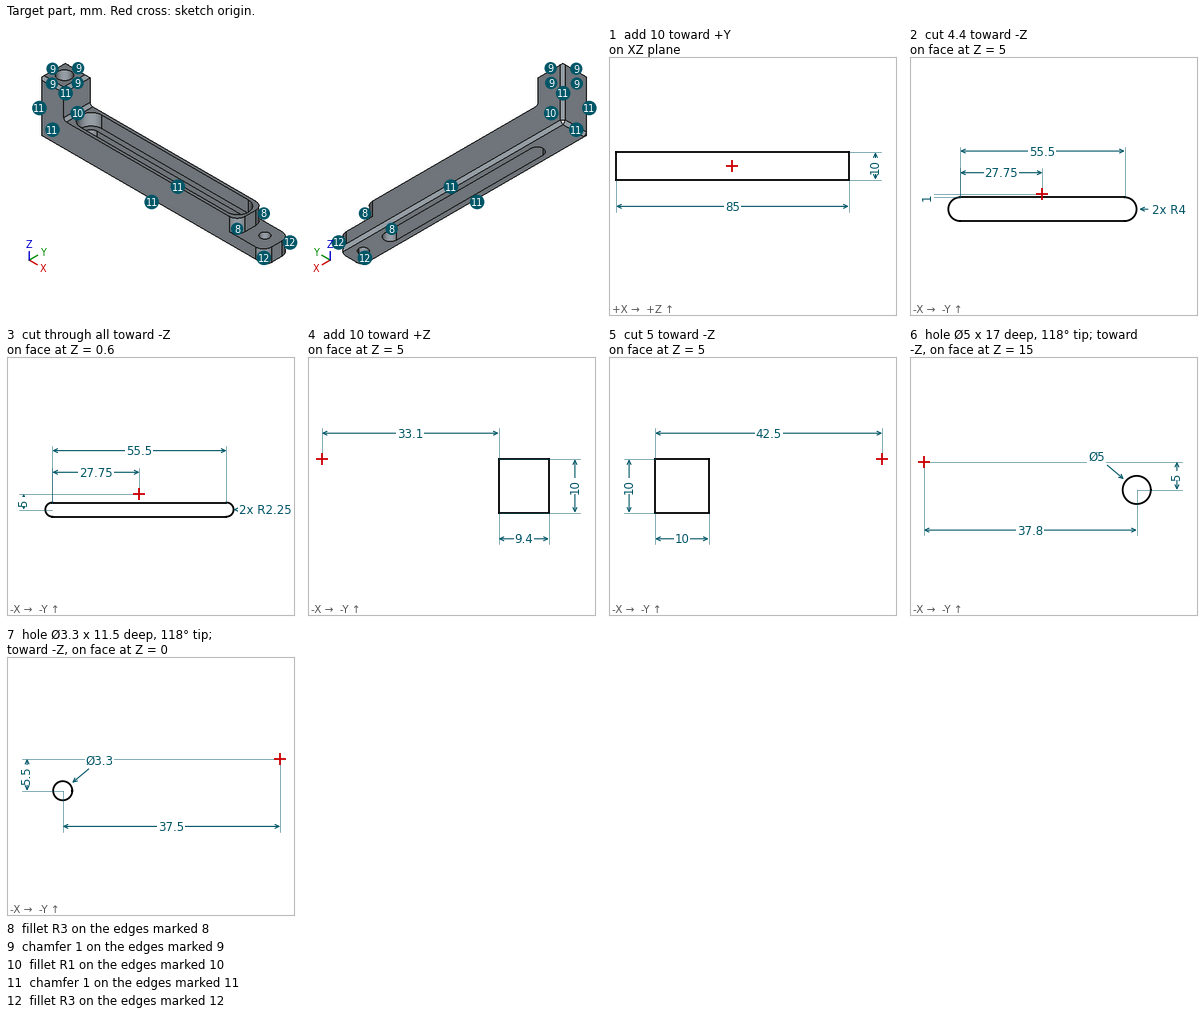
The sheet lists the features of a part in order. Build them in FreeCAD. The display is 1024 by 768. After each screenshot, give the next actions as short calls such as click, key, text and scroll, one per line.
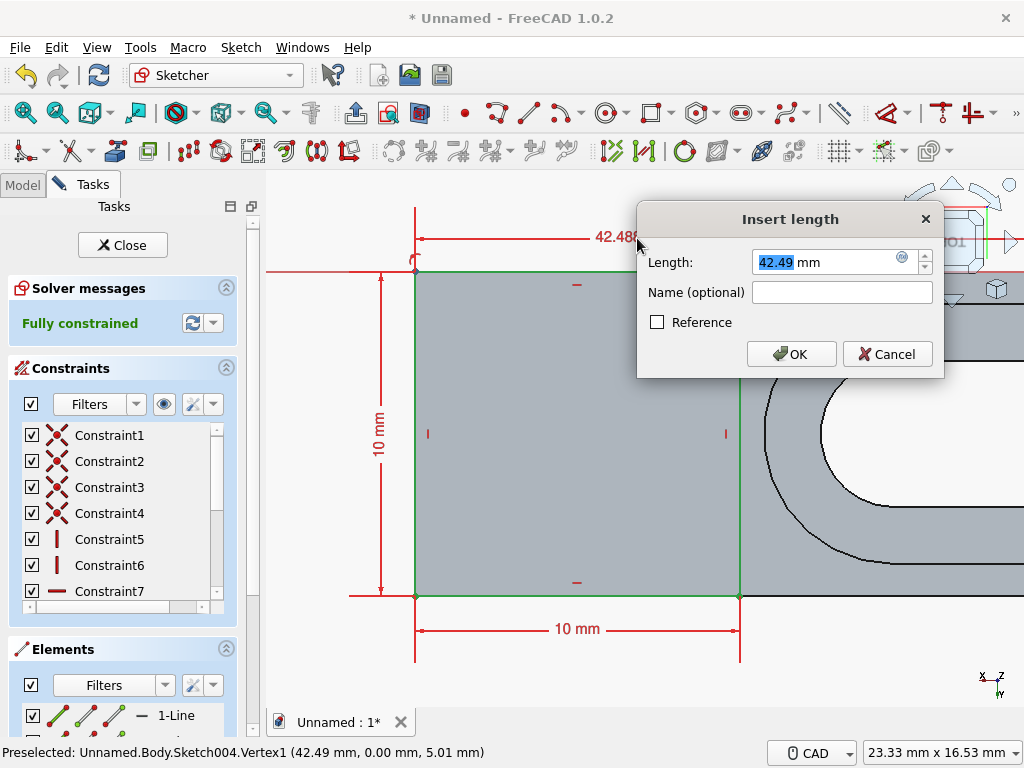
text(42.5)
key(Return)
key(Escape)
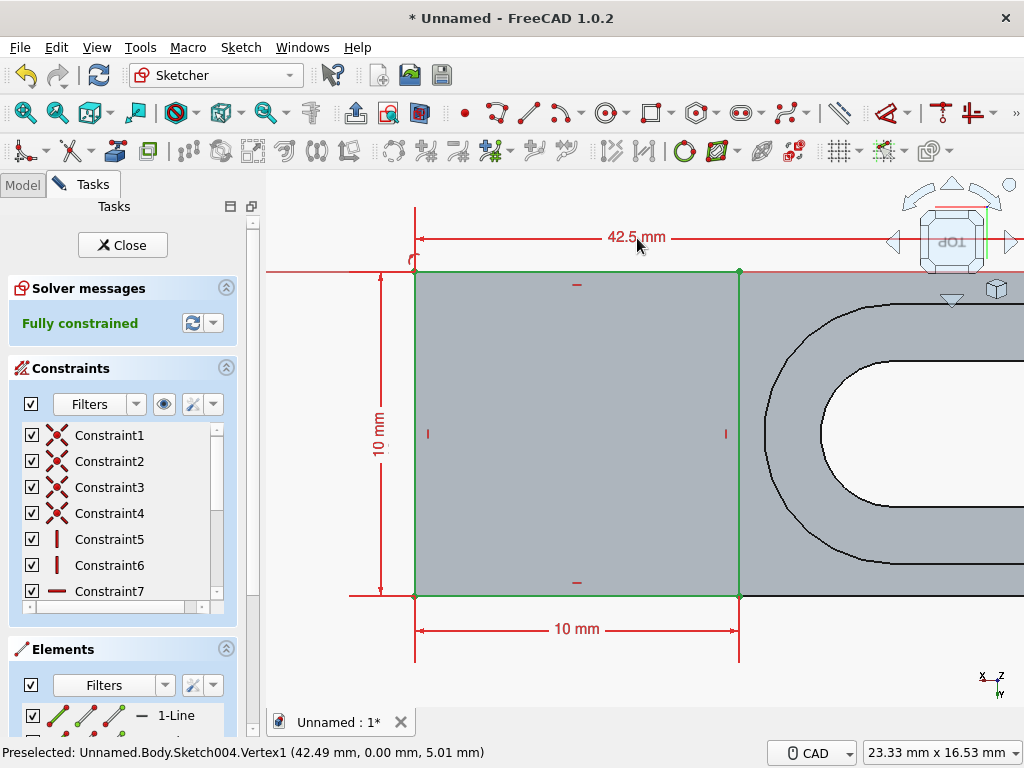
click(123, 245)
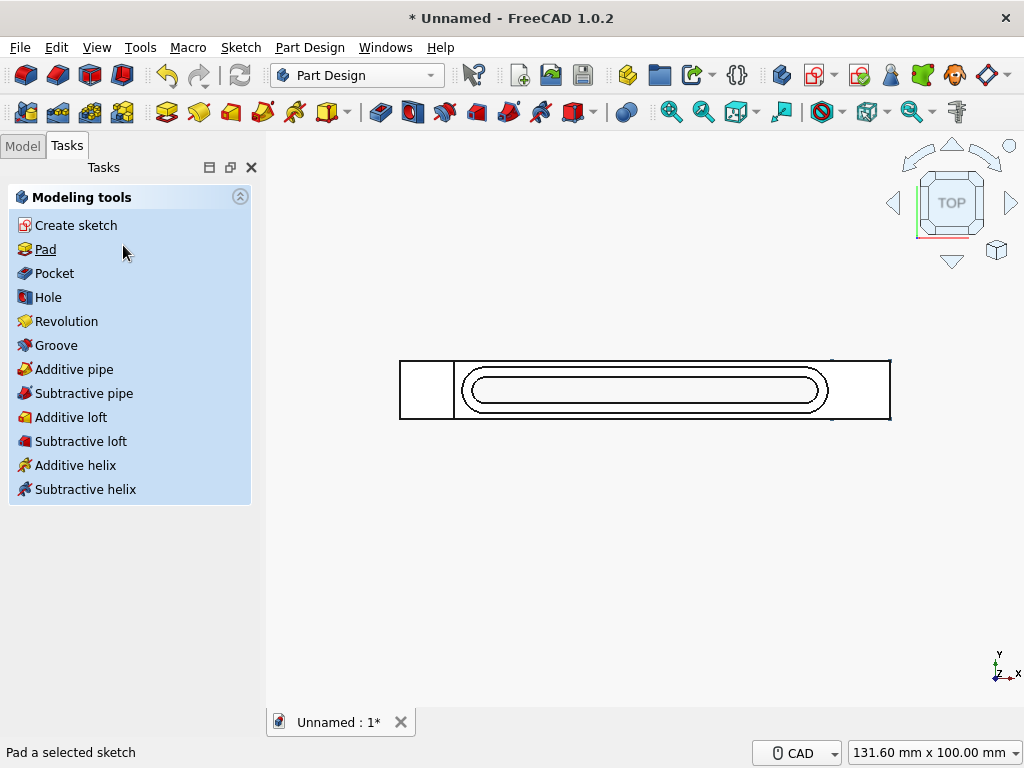
click(382, 112)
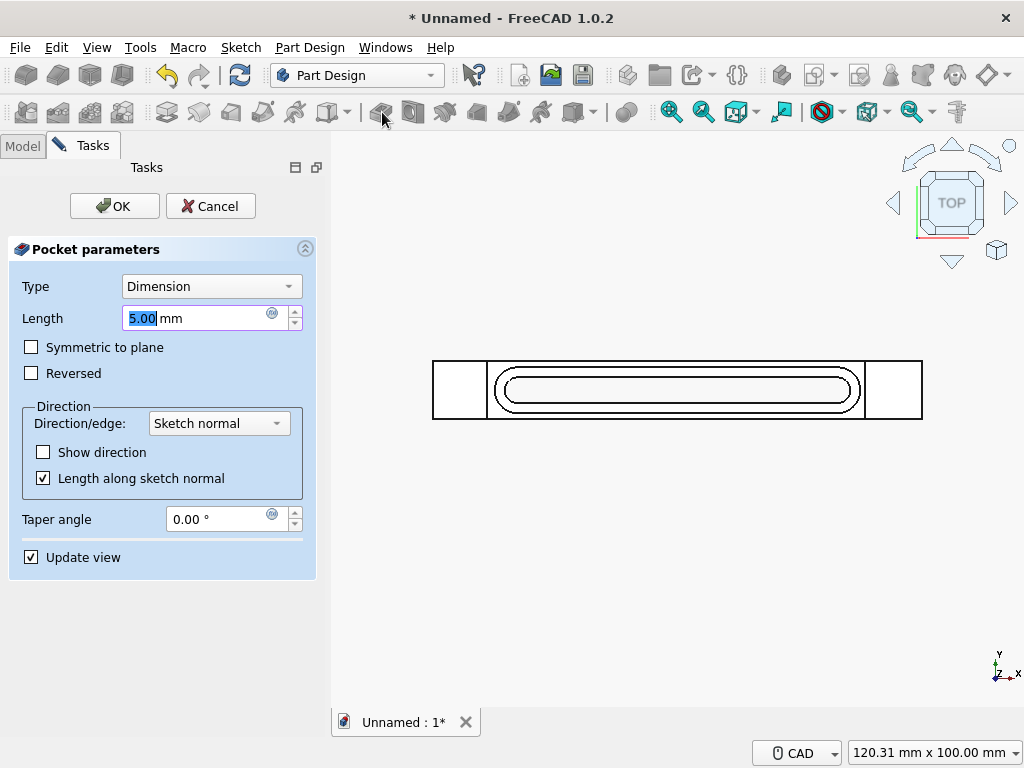
text(5)
key(Tab)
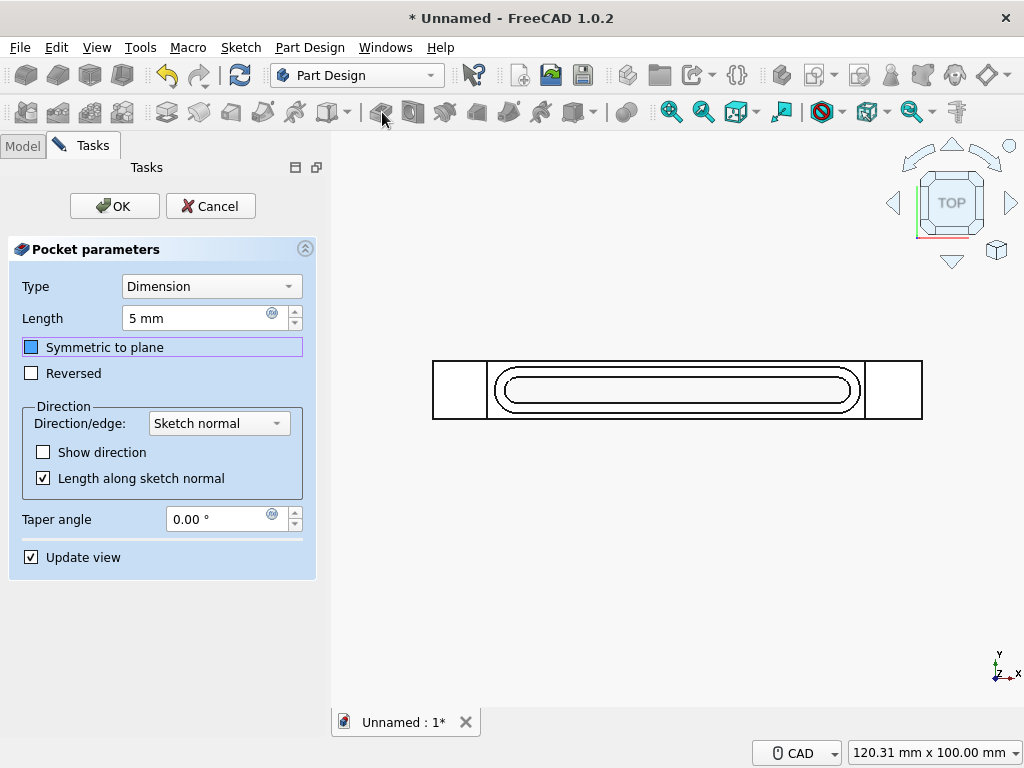
click(115, 206)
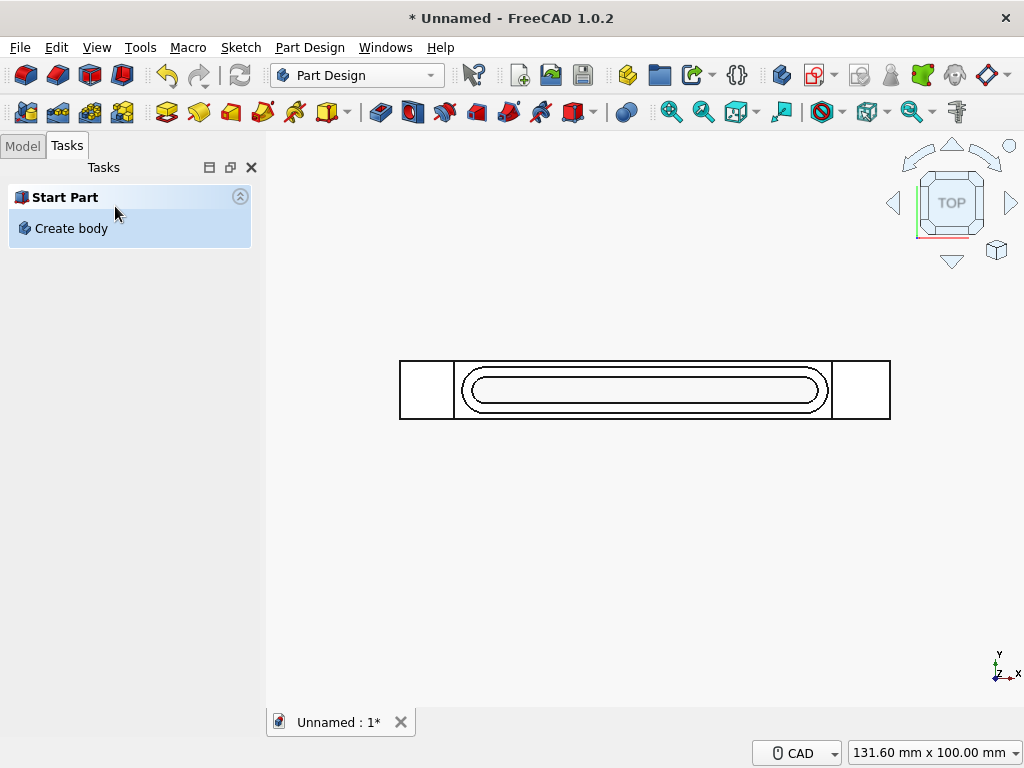
click(427, 389)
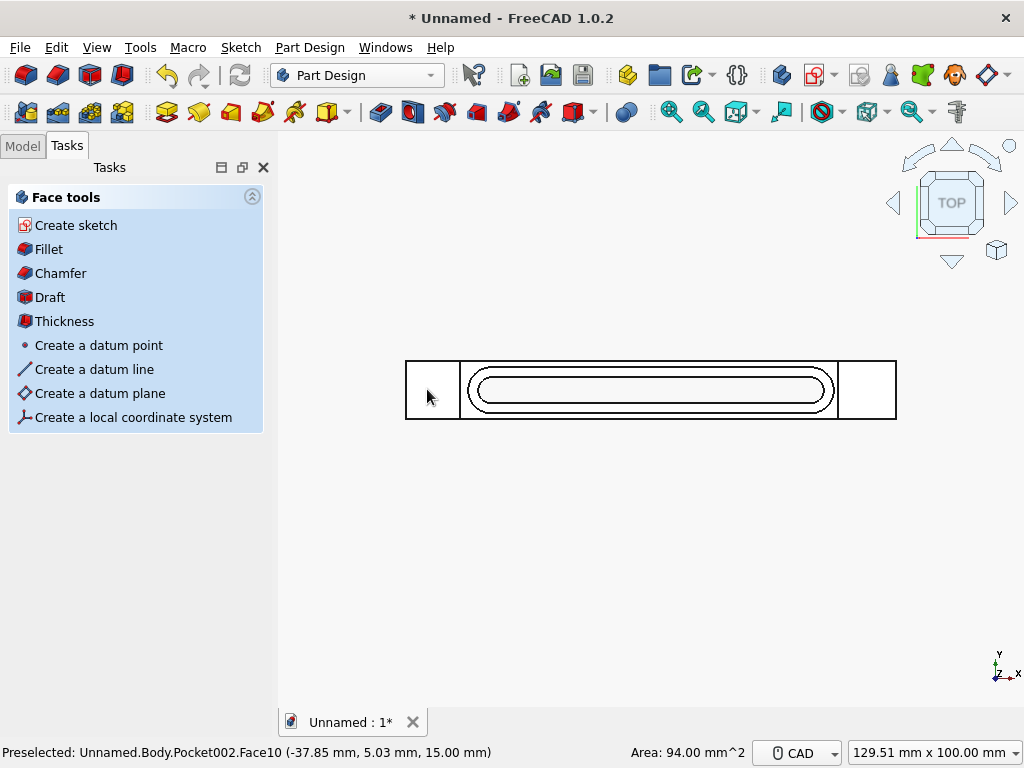
click(814, 76)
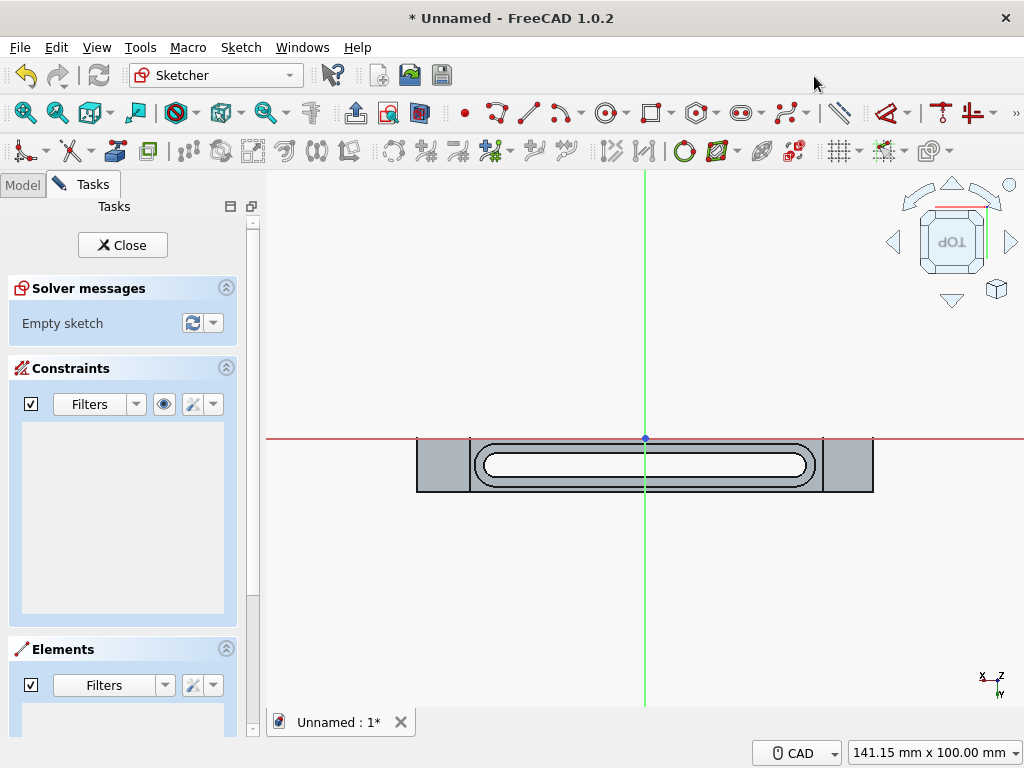
scroll(576, 438, down, 5)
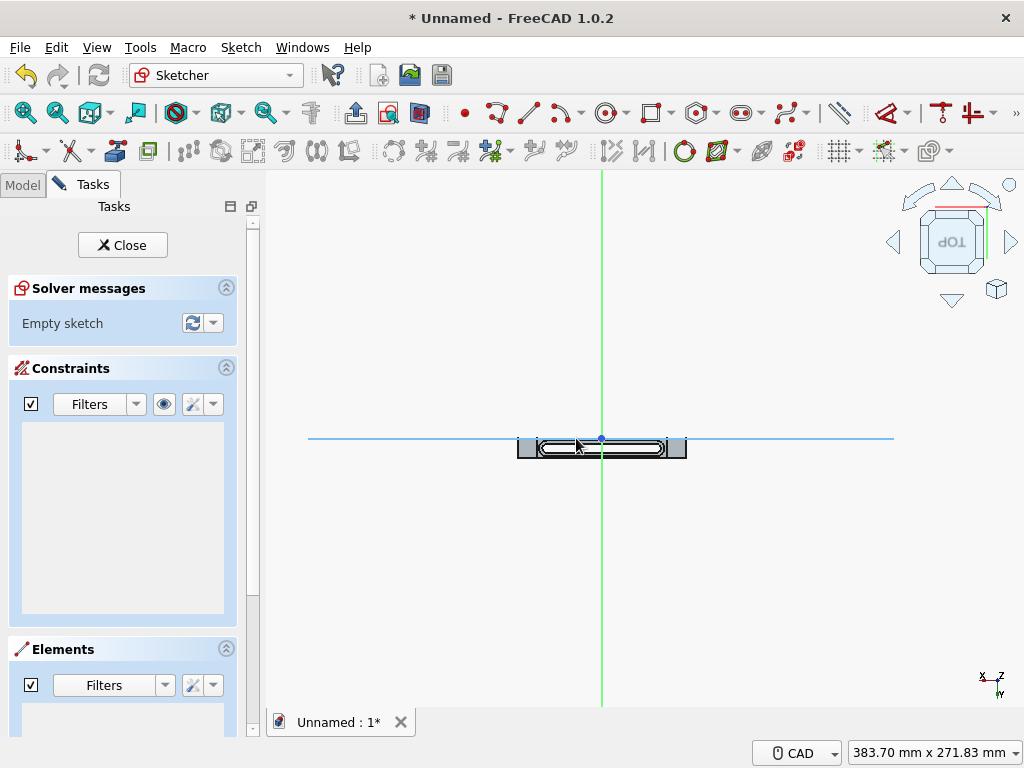
scroll(682, 449, up, 15)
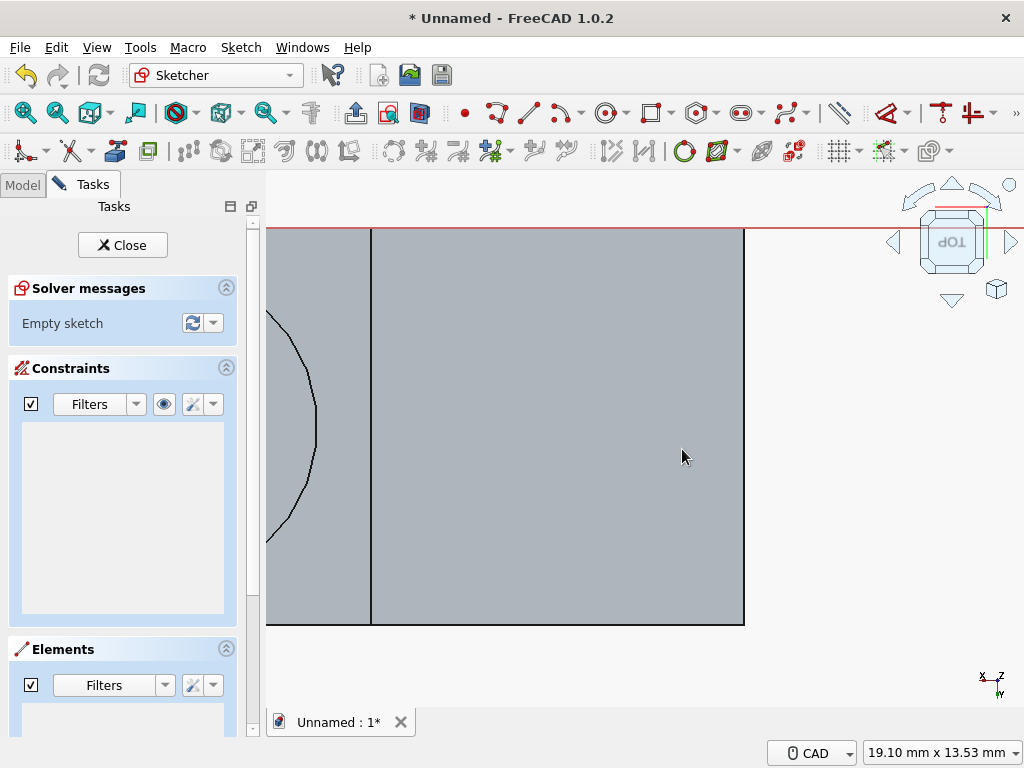
scroll(534, 412, up, 3)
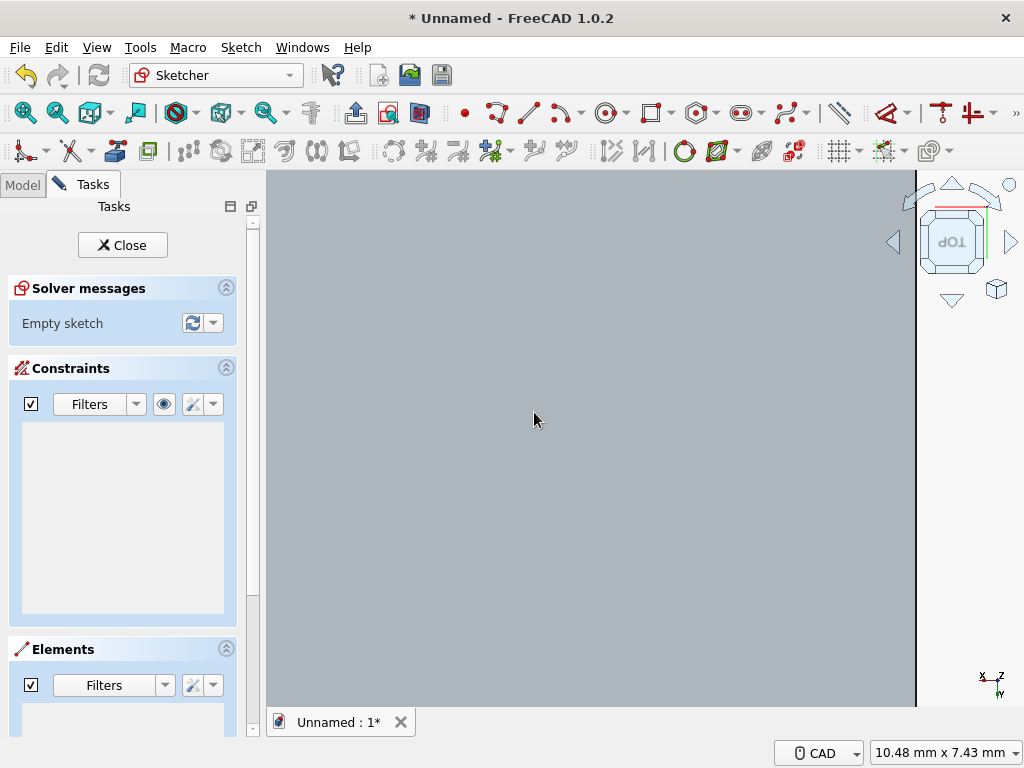
key(g)
key(c)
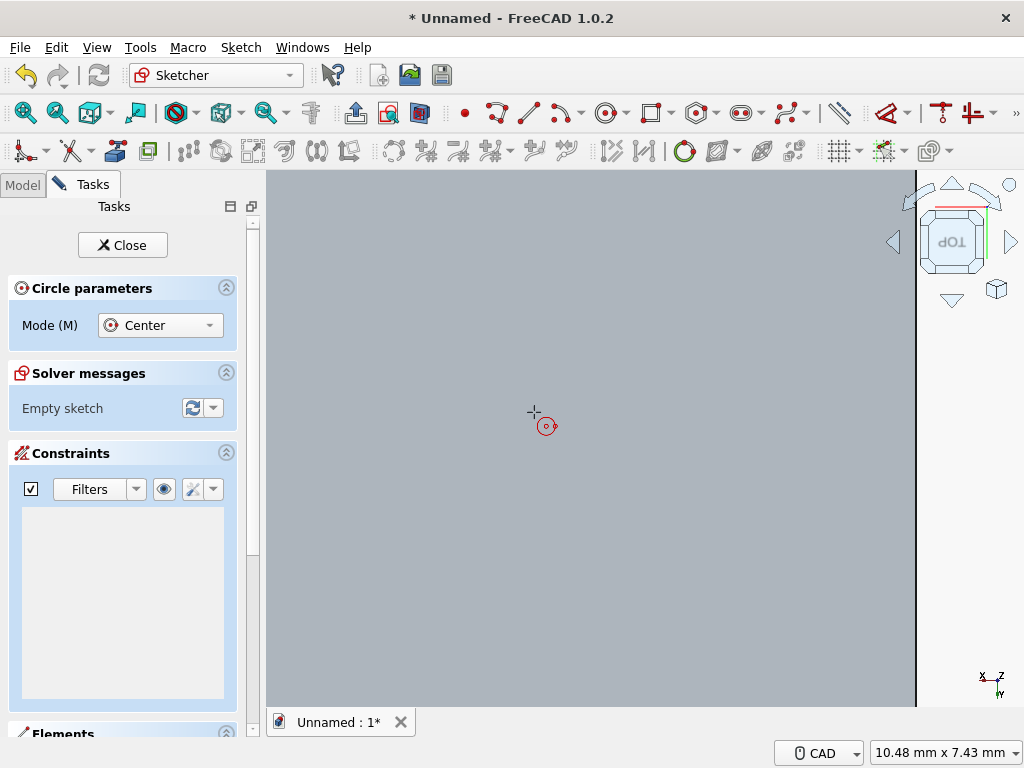
click(576, 438)
click(704, 310)
key(Escape)